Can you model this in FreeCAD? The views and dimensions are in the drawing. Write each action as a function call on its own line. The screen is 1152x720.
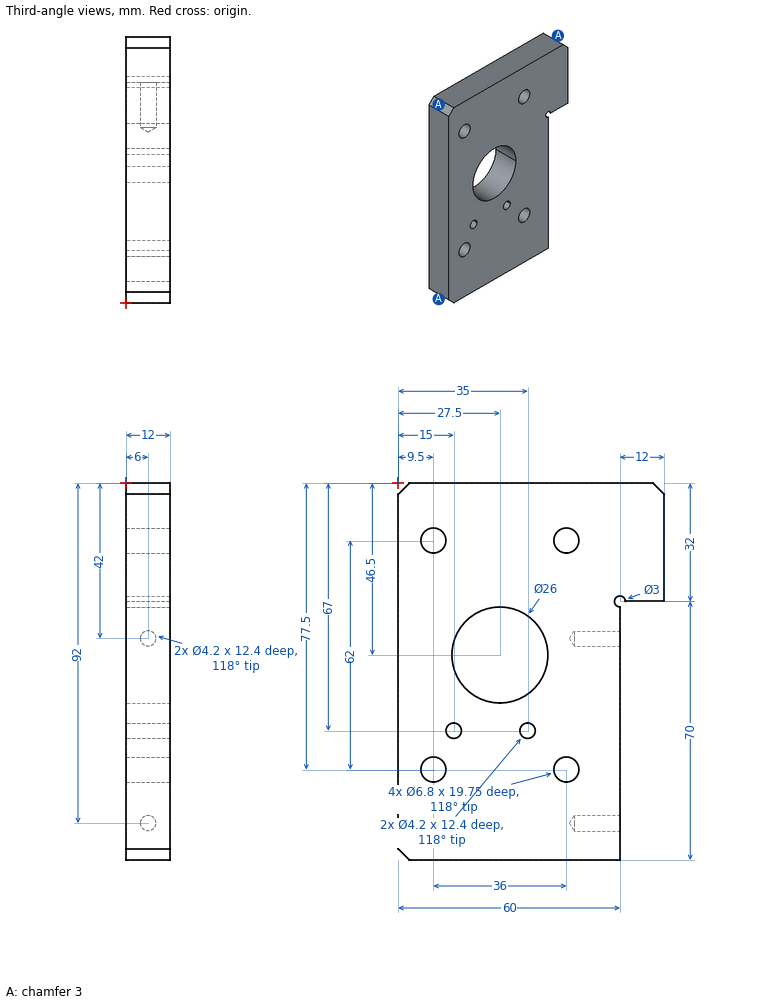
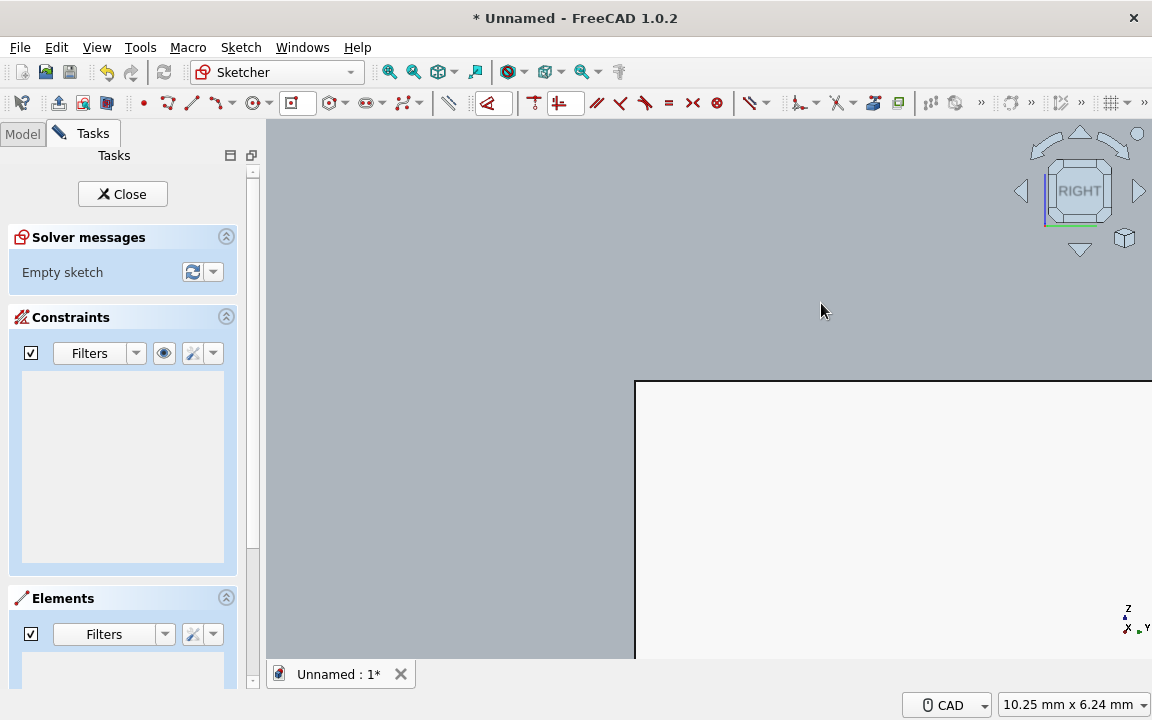
click(254, 104)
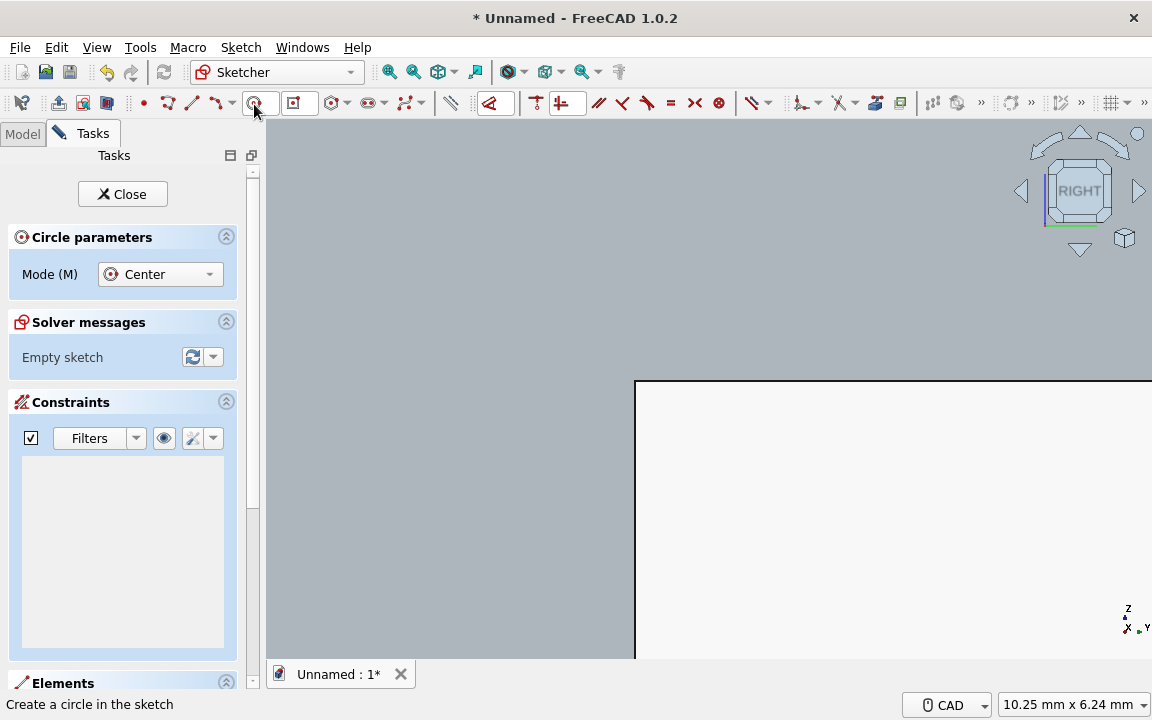
click(635, 381)
move(727, 289)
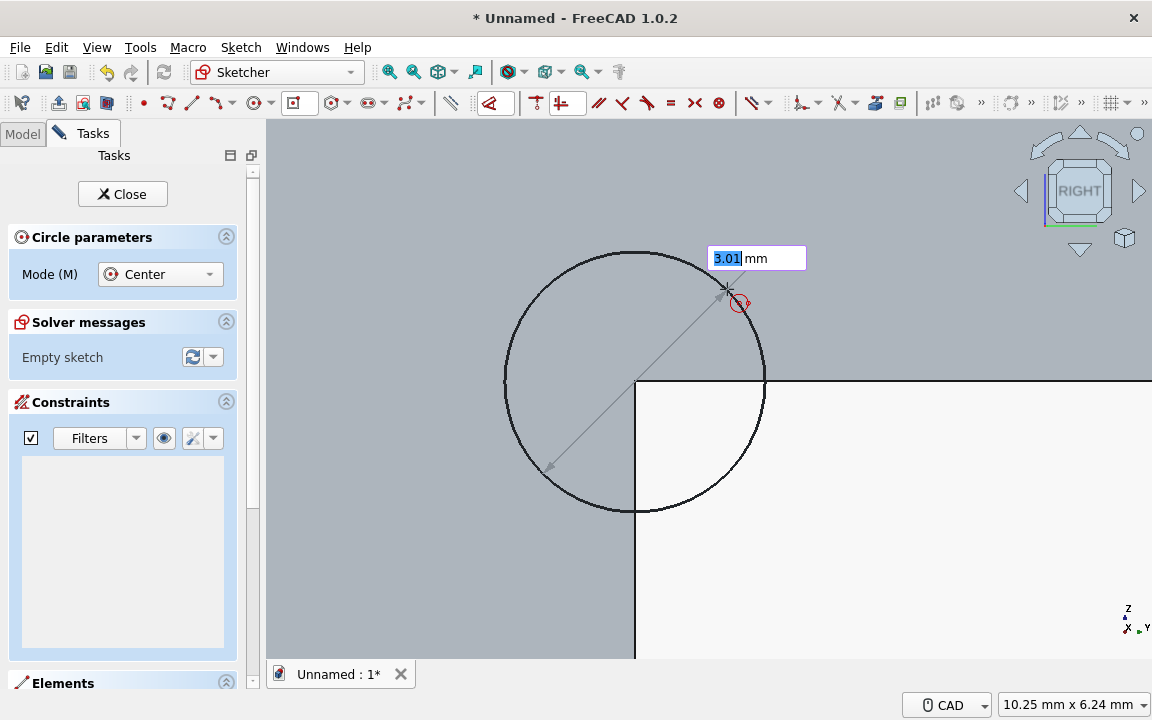
text(3)
key(Return)
key(Escape)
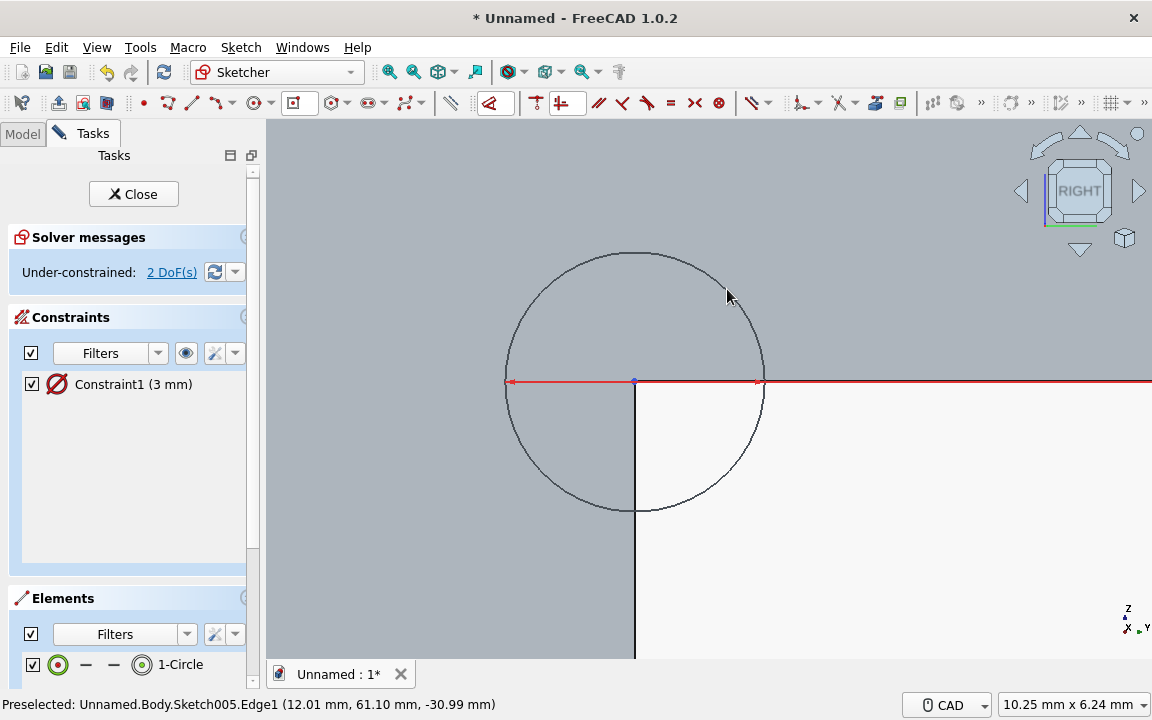
click(635, 382)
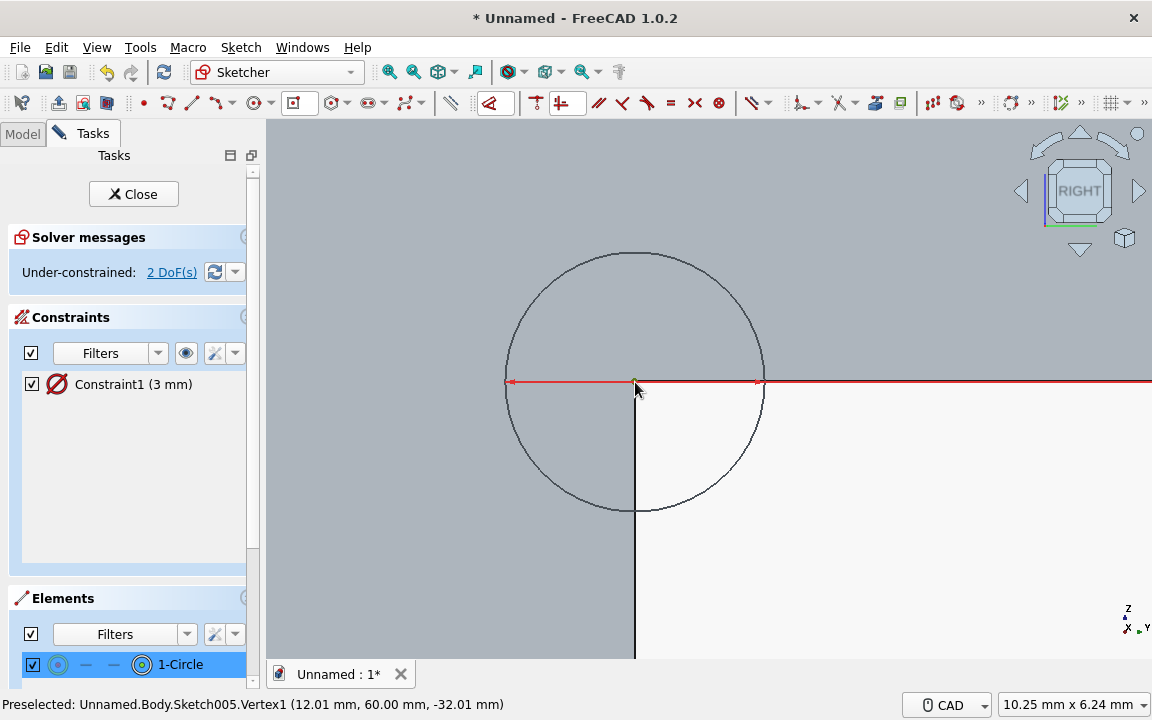
click(508, 104)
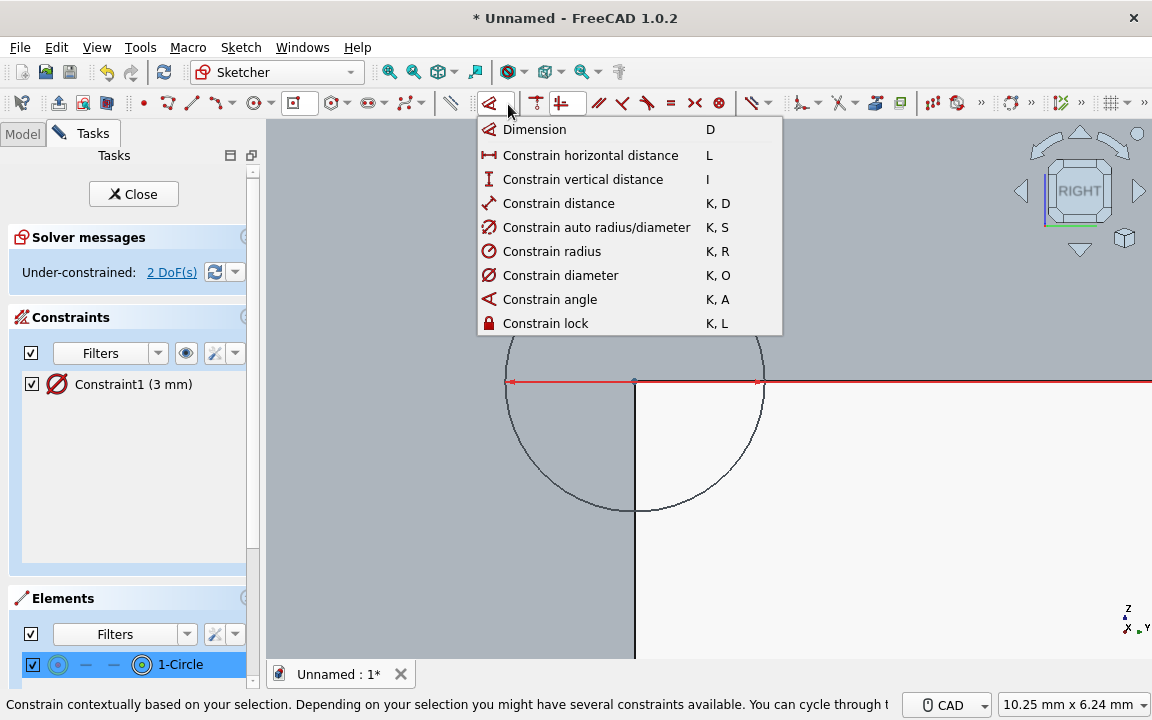
click(630, 155)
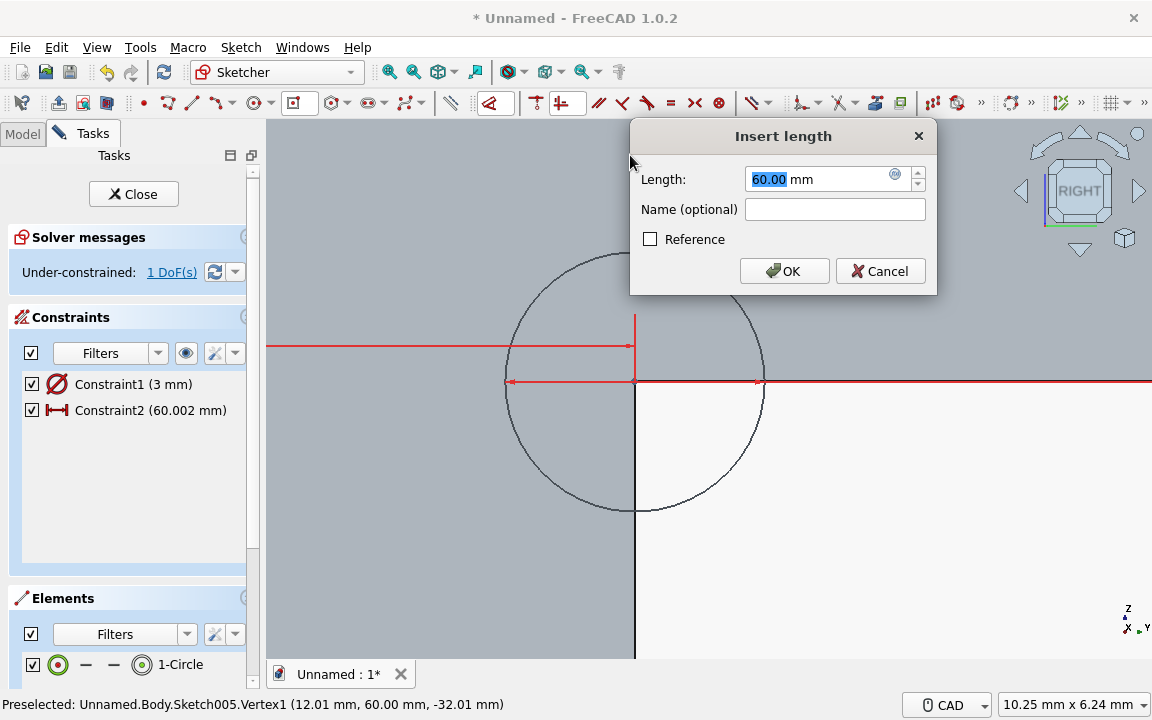
text(60)
key(Return)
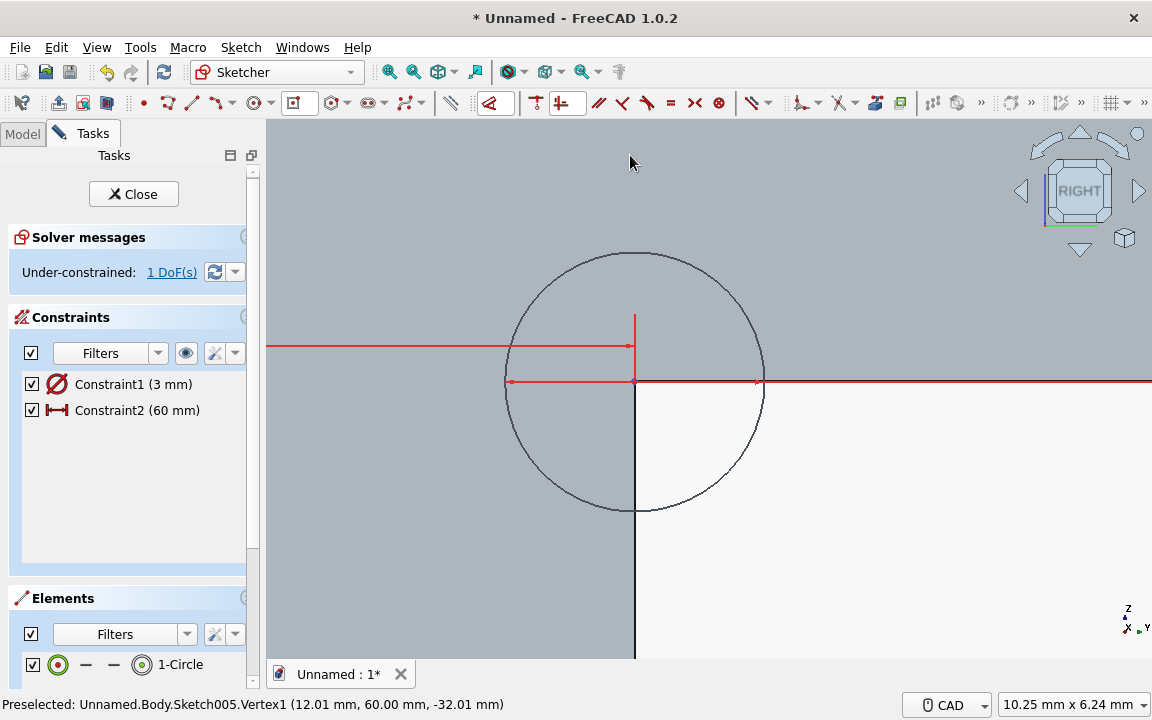
click(635, 382)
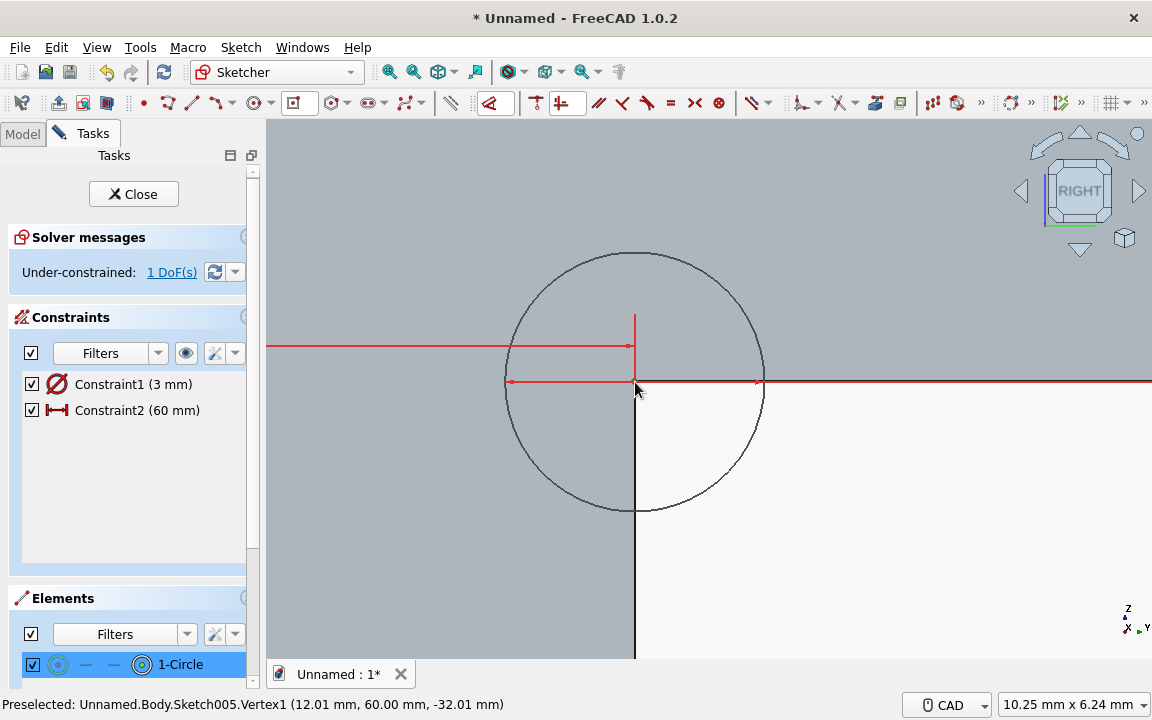
click(508, 104)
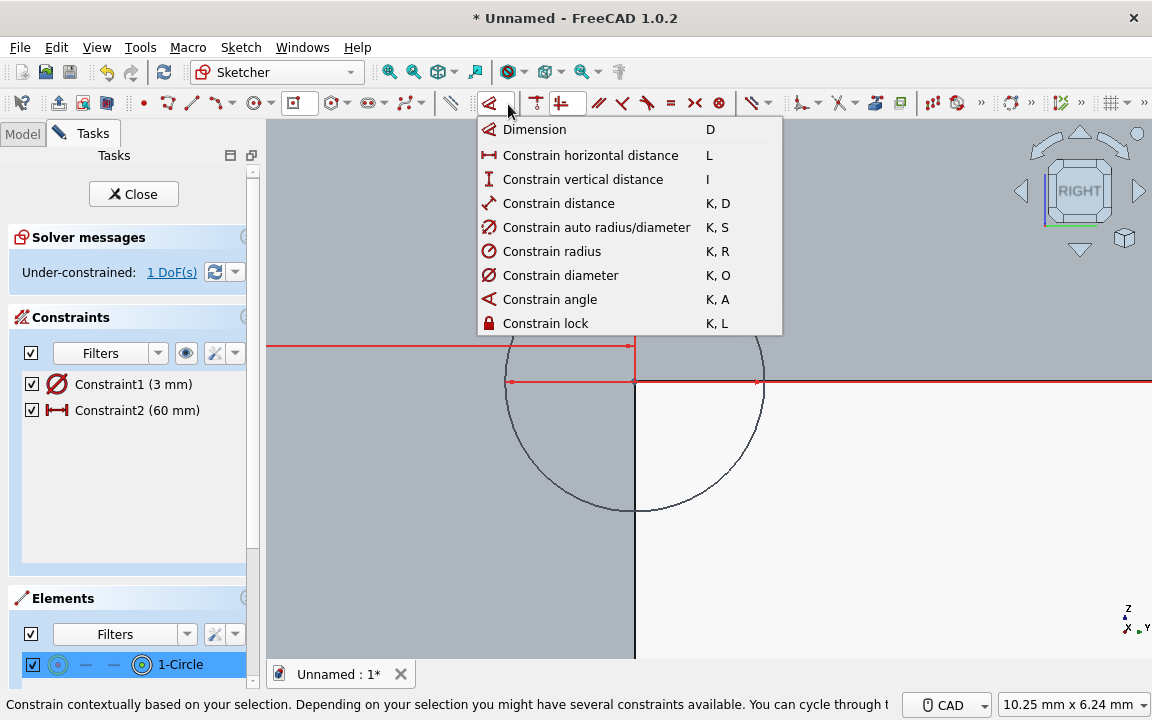
click(630, 179)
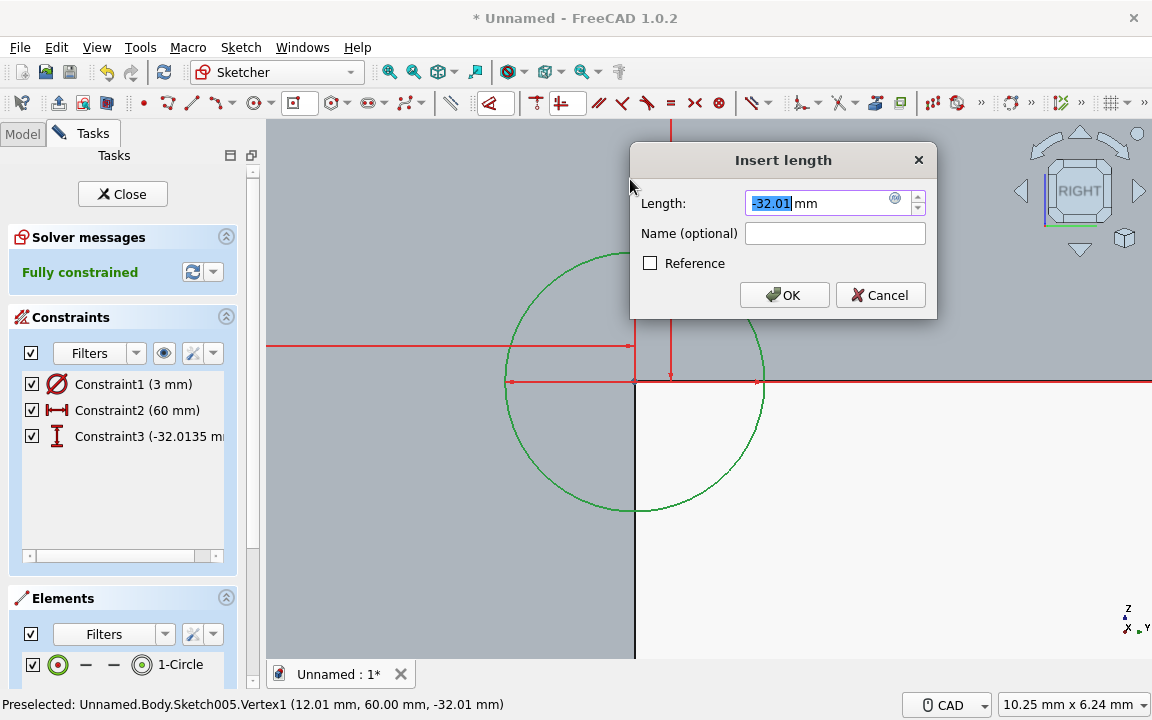
text(-32)
key(Return)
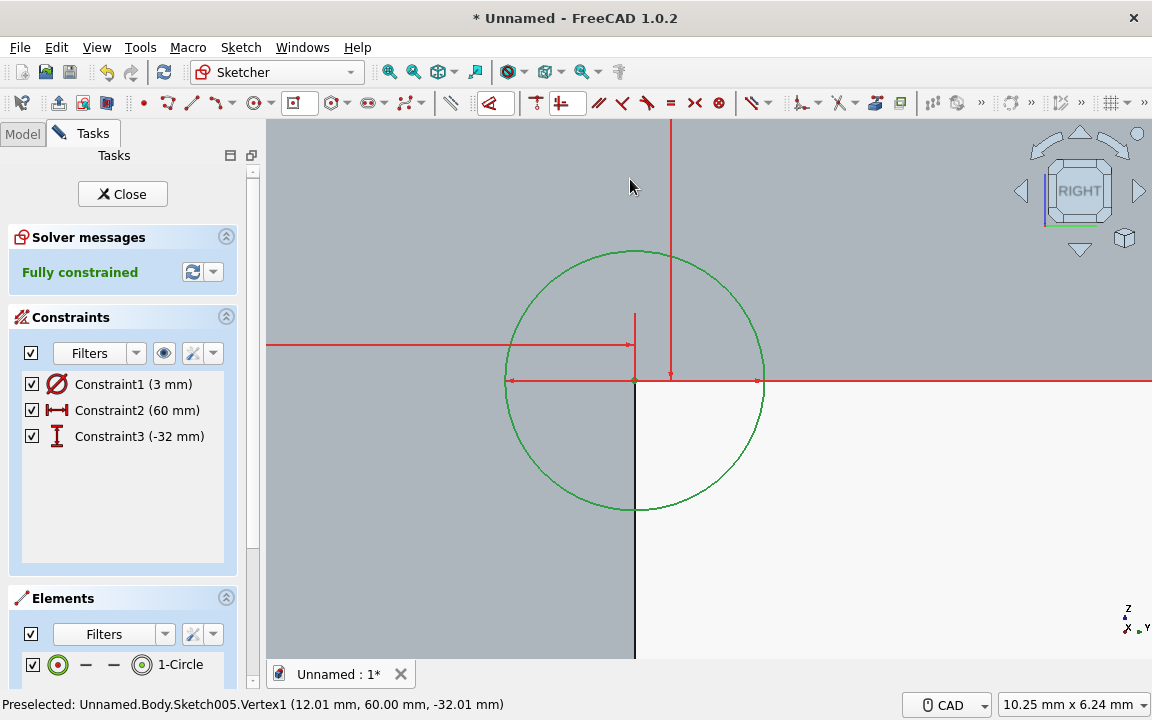
click(123, 194)